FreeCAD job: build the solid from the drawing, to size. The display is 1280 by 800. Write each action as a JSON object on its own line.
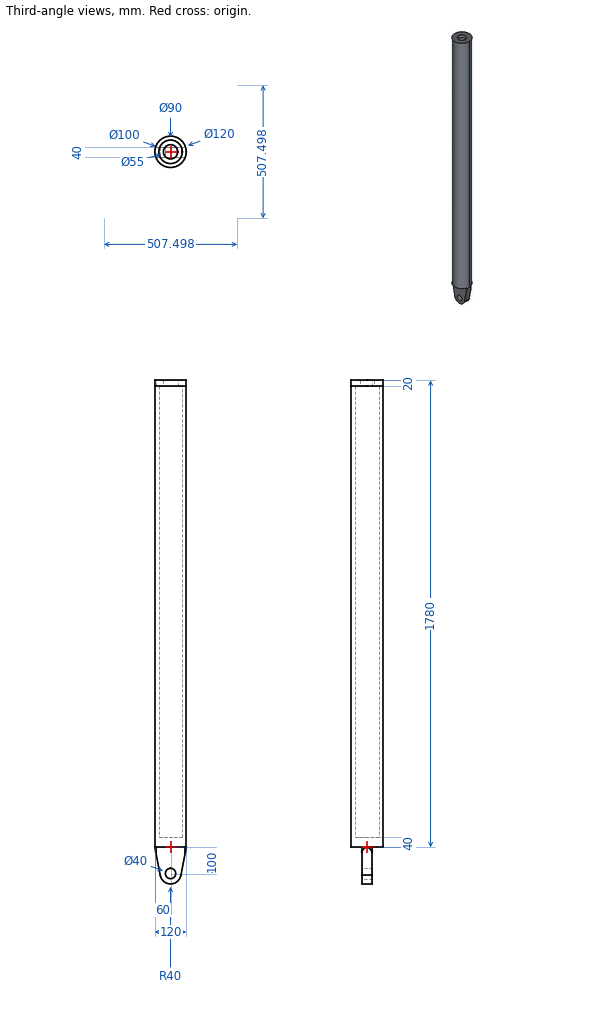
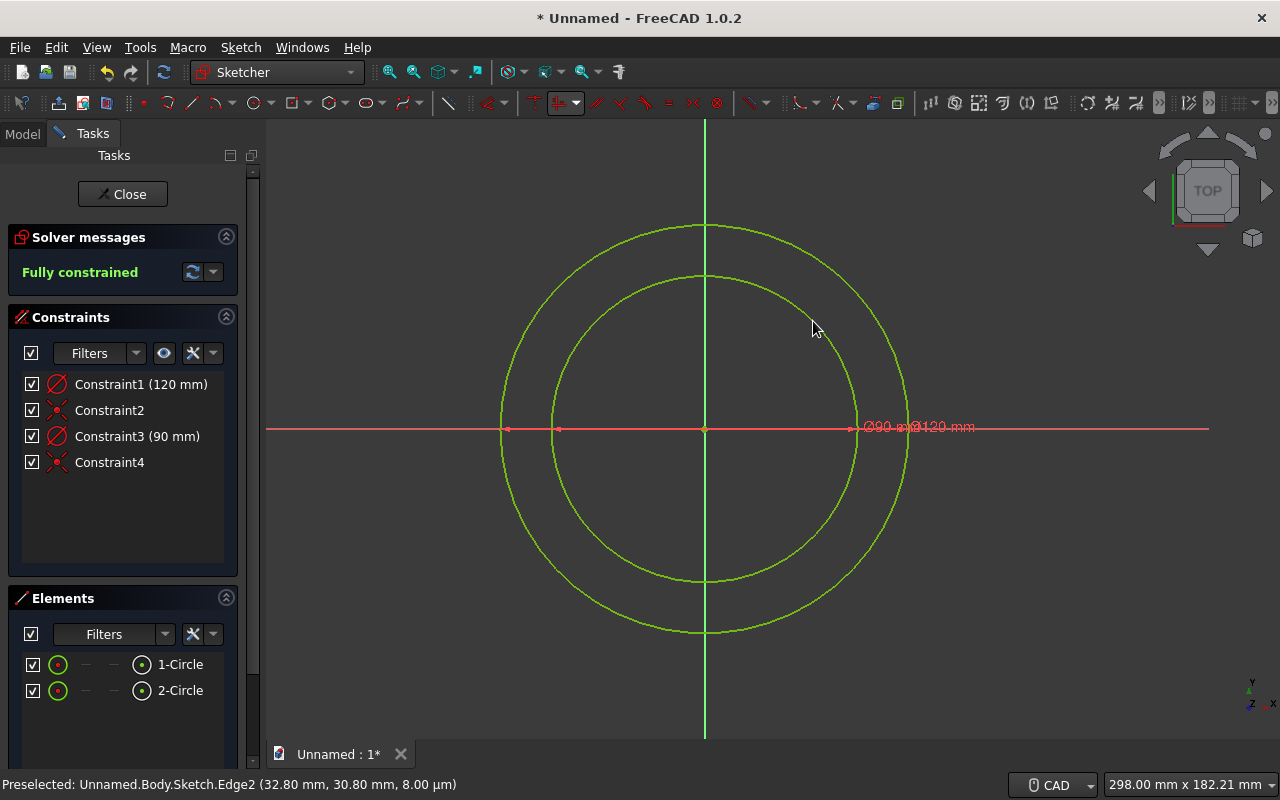
{"action": "left_click", "coordinate": [123, 194]}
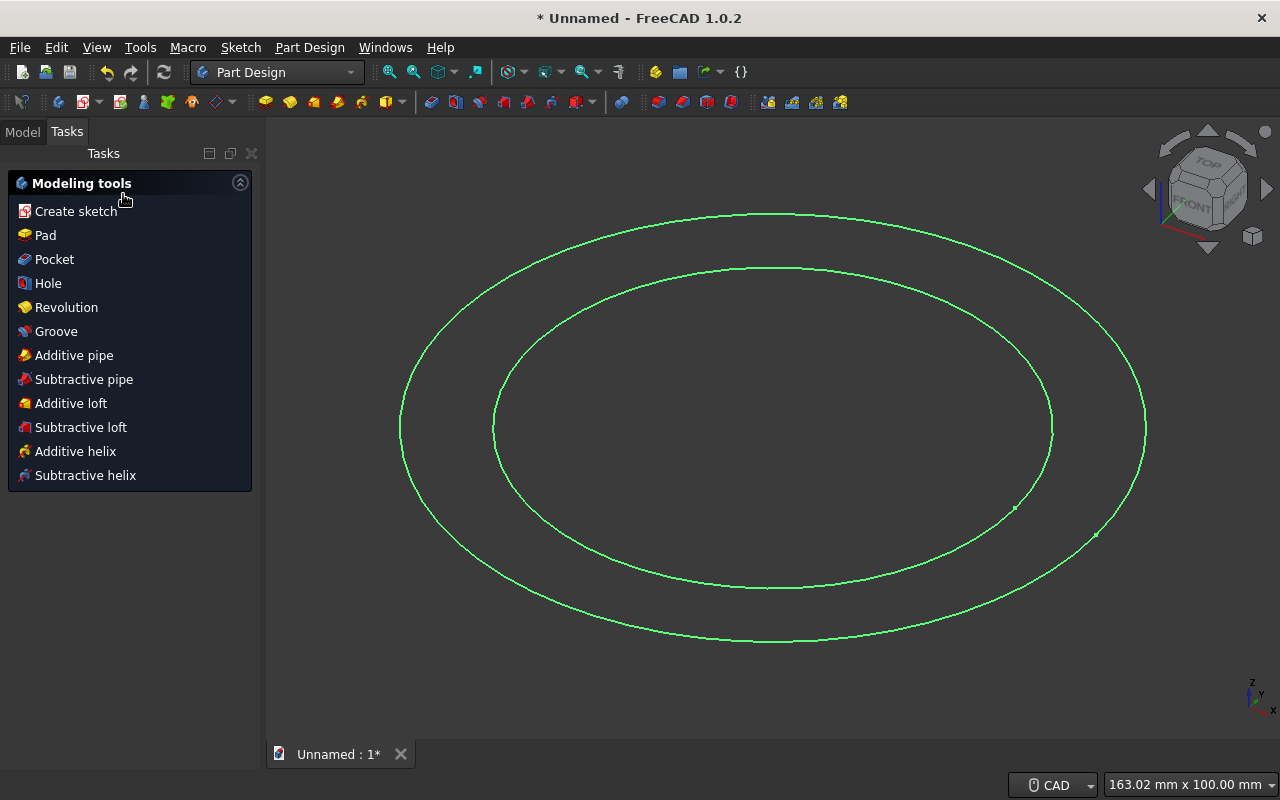
{"action": "left_click", "coordinate": [266, 102]}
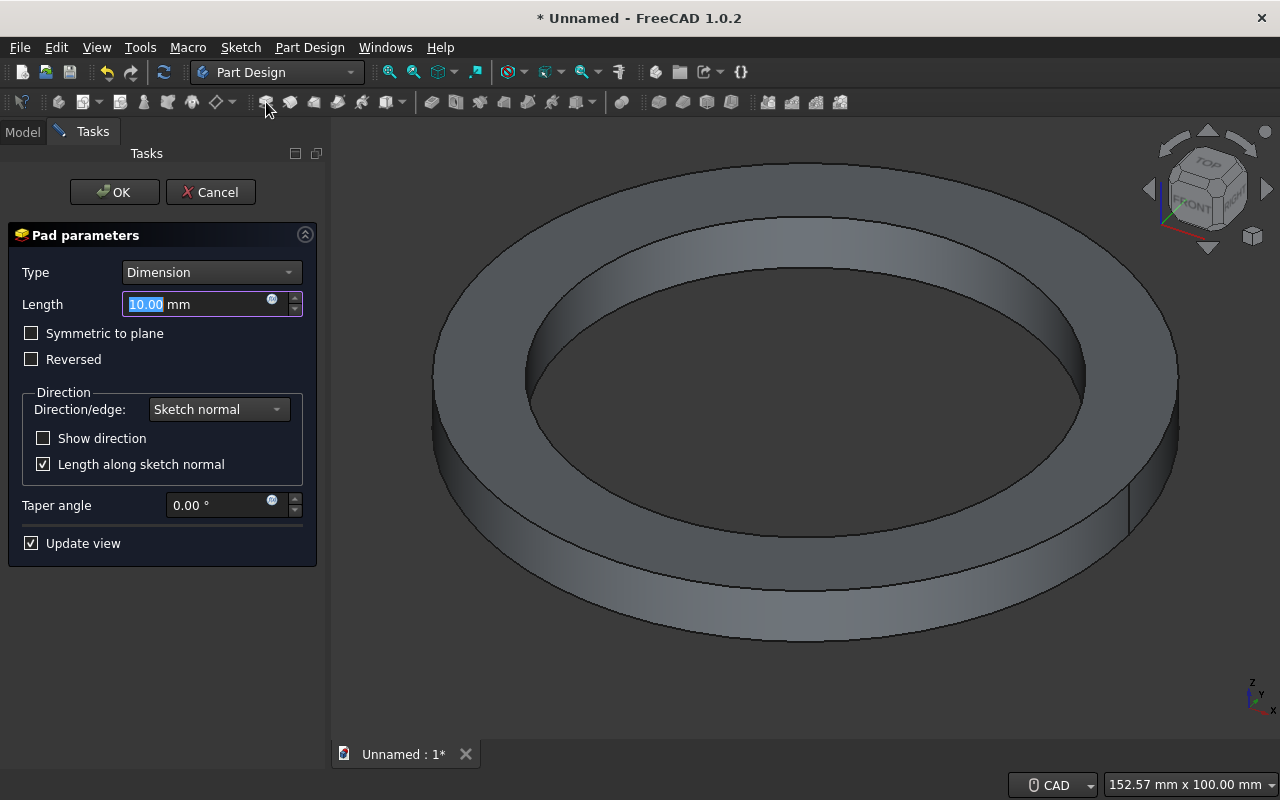
{"action": "type", "text": "1780"}
{"action": "key", "text": "Tab"}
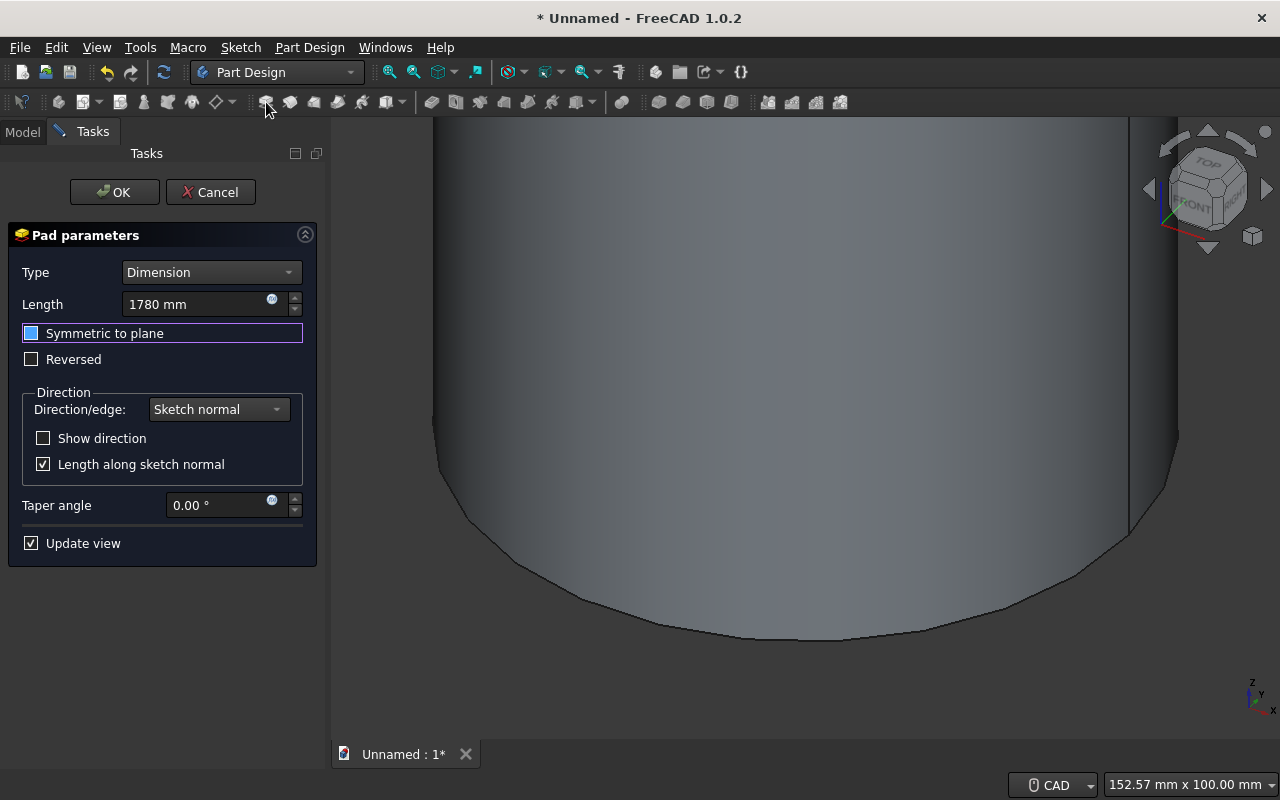
{"action": "left_click", "coordinate": [115, 192]}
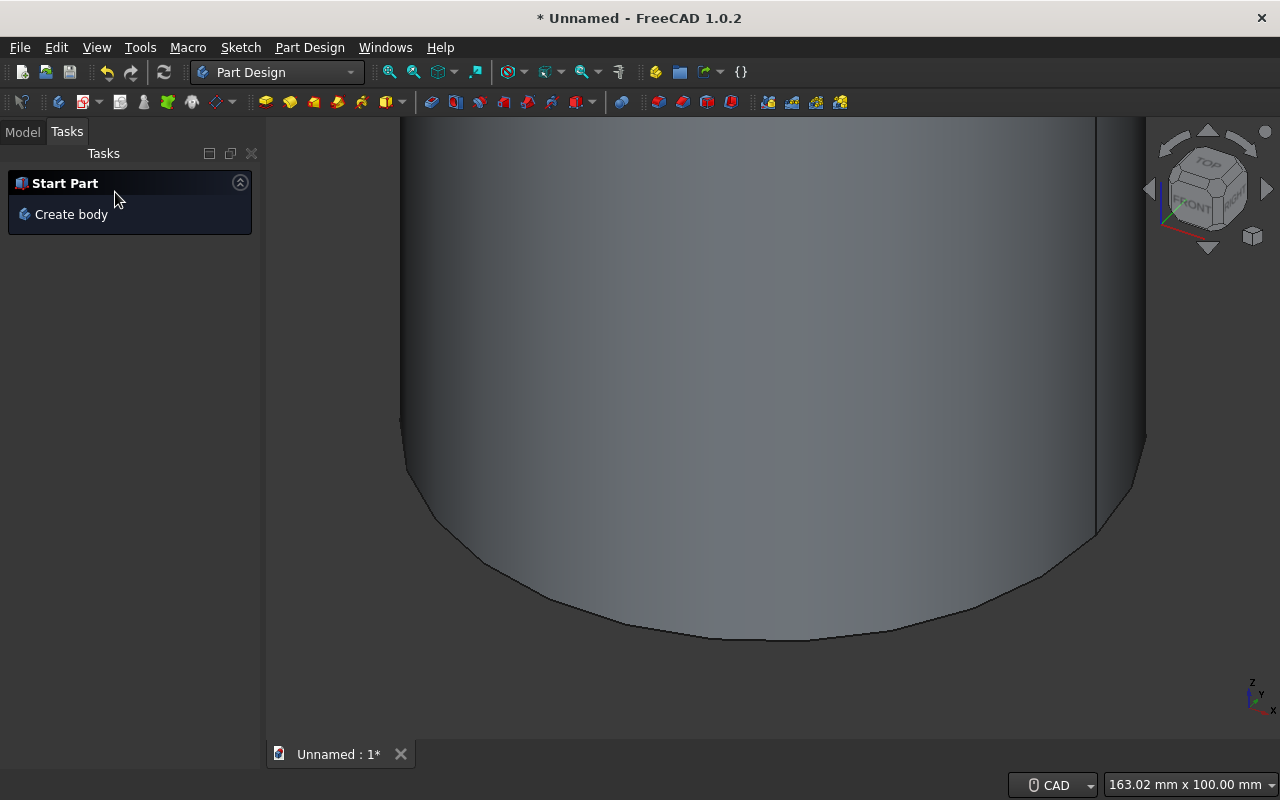
{"action": "key", "text": "v f"}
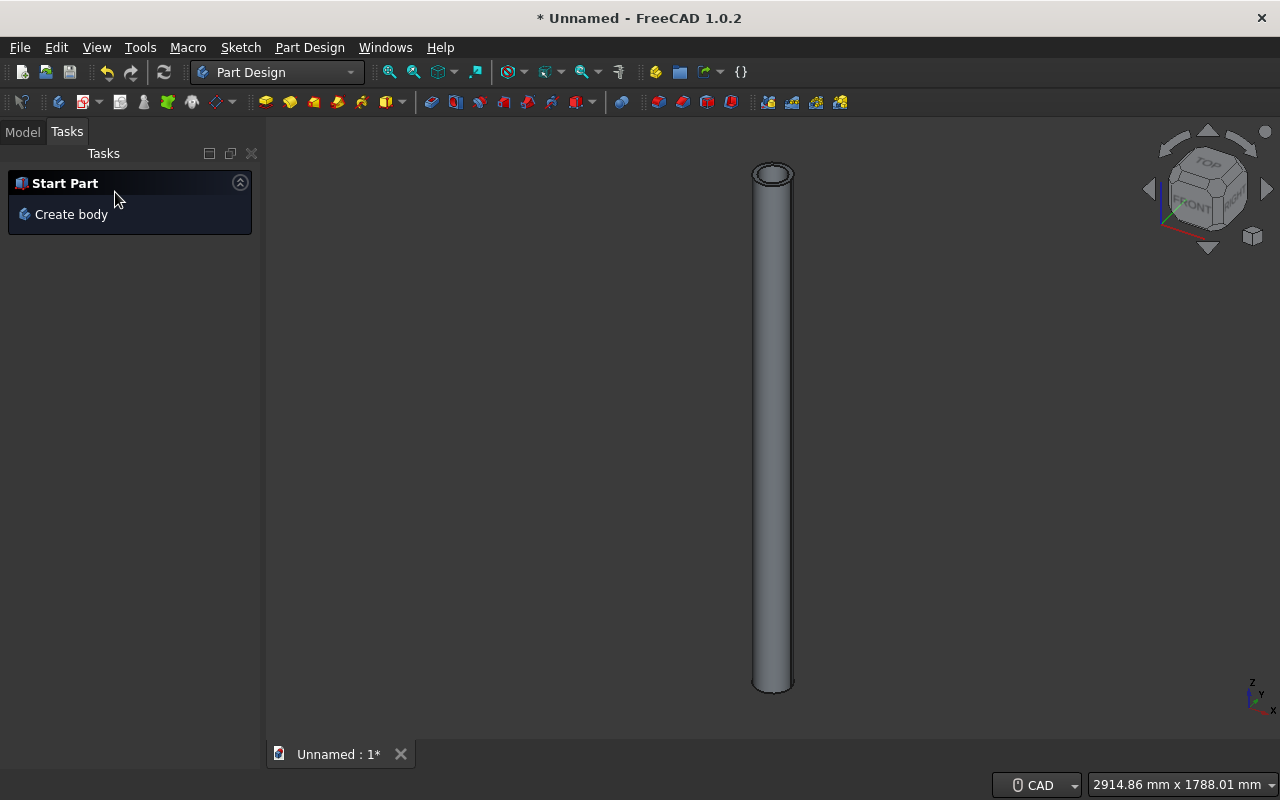
{"action": "left_click", "coordinate": [84, 102]}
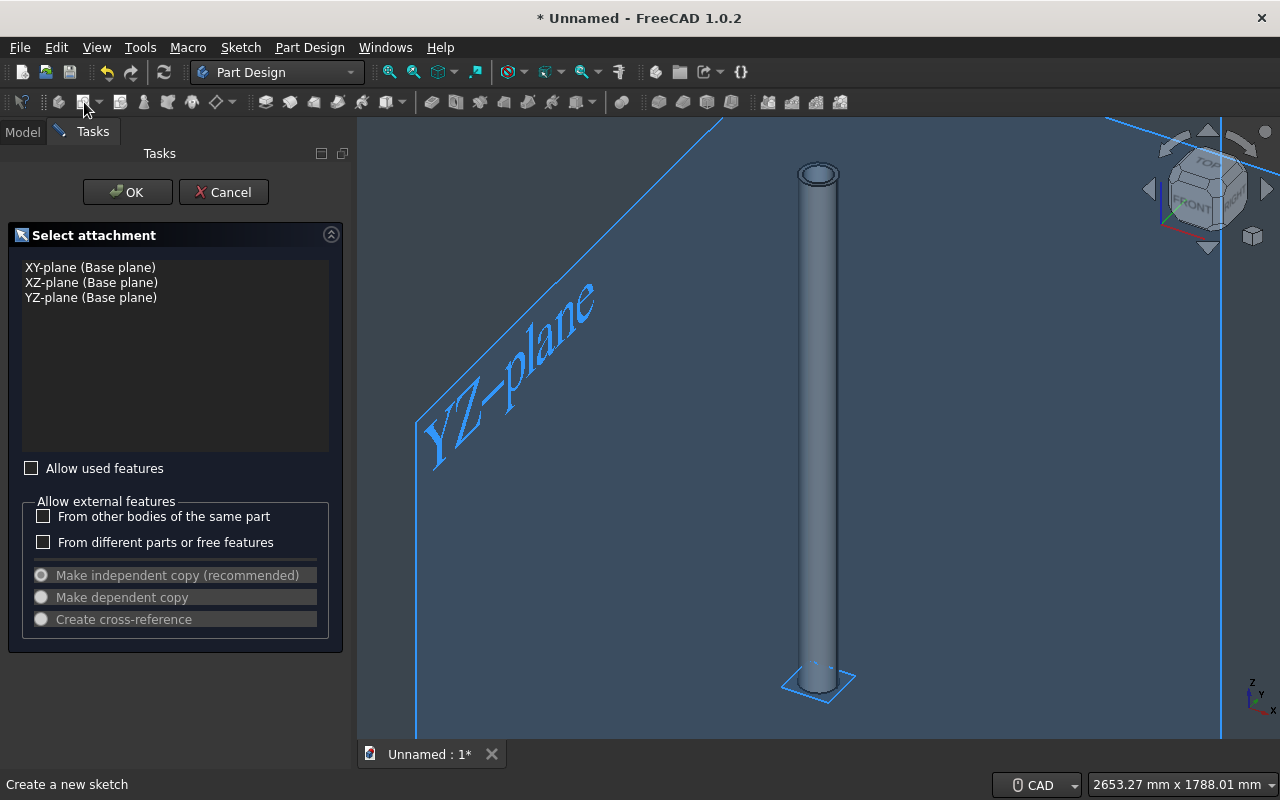
{"action": "left_click", "coordinate": [82, 282]}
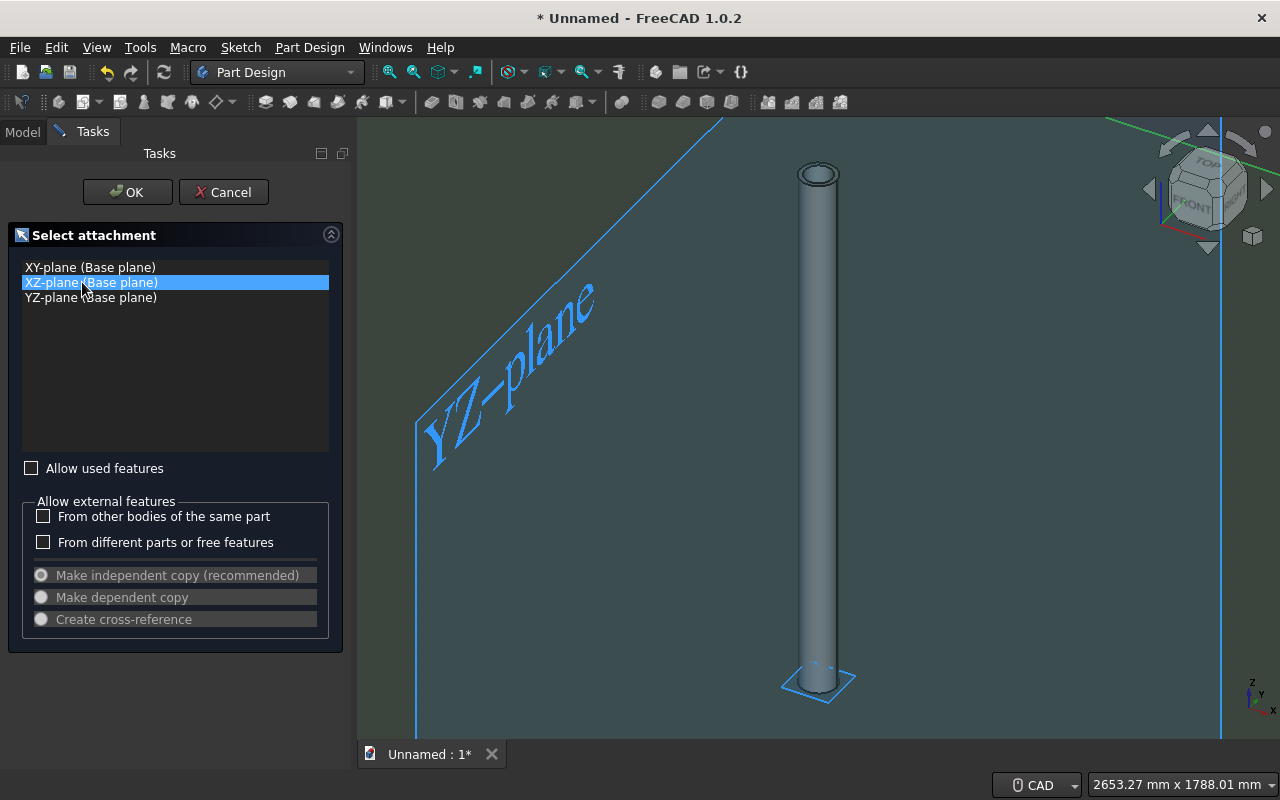
{"action": "left_click", "coordinate": [128, 192]}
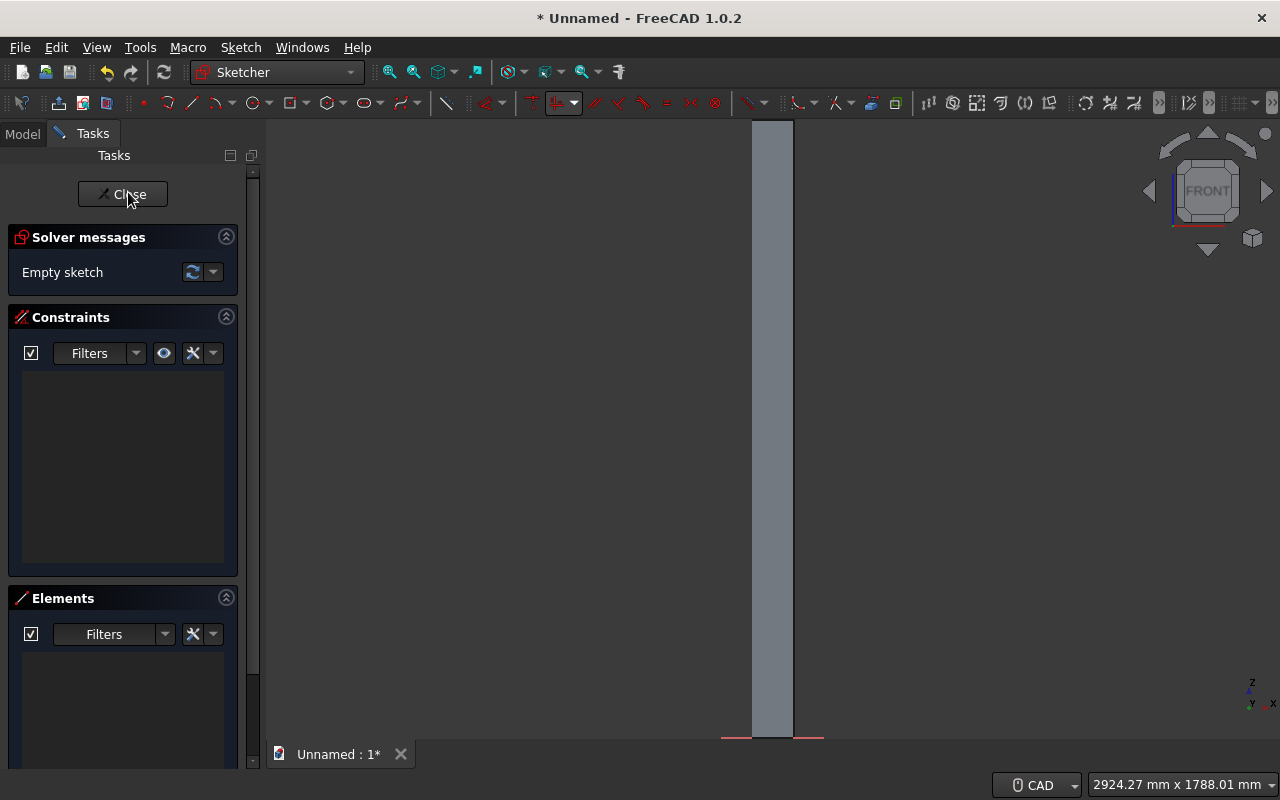
{"action": "key", "text": "q s"}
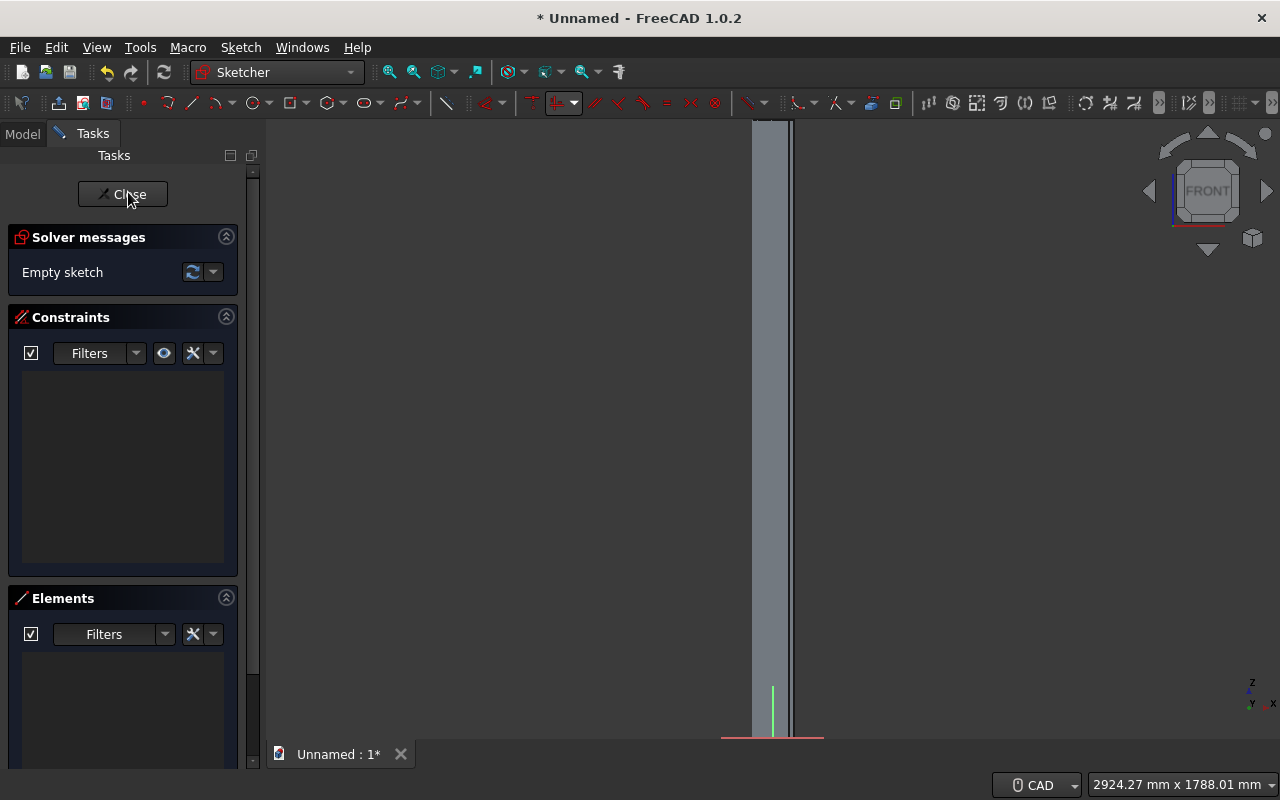
{"action": "scroll", "coordinate": [704, 429], "scroll_direction": "down", "scroll_amount": 5}